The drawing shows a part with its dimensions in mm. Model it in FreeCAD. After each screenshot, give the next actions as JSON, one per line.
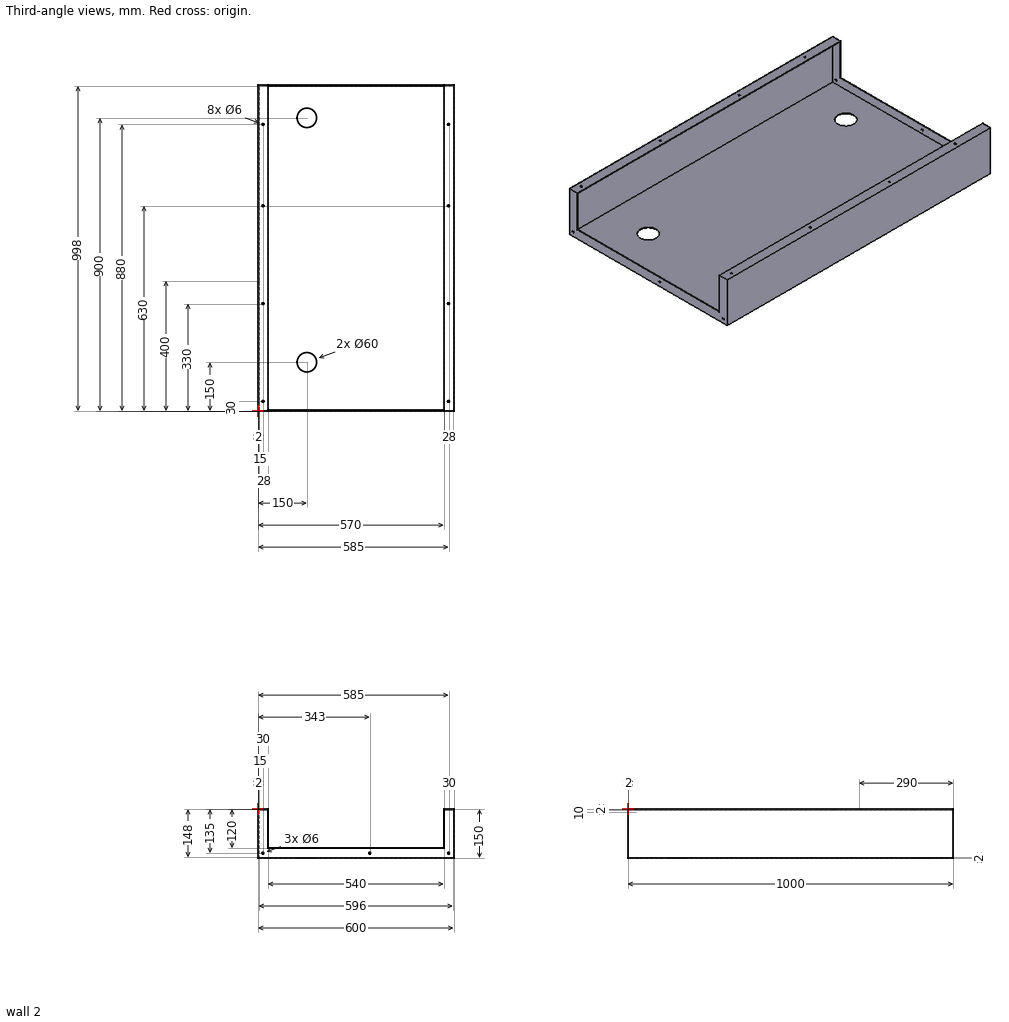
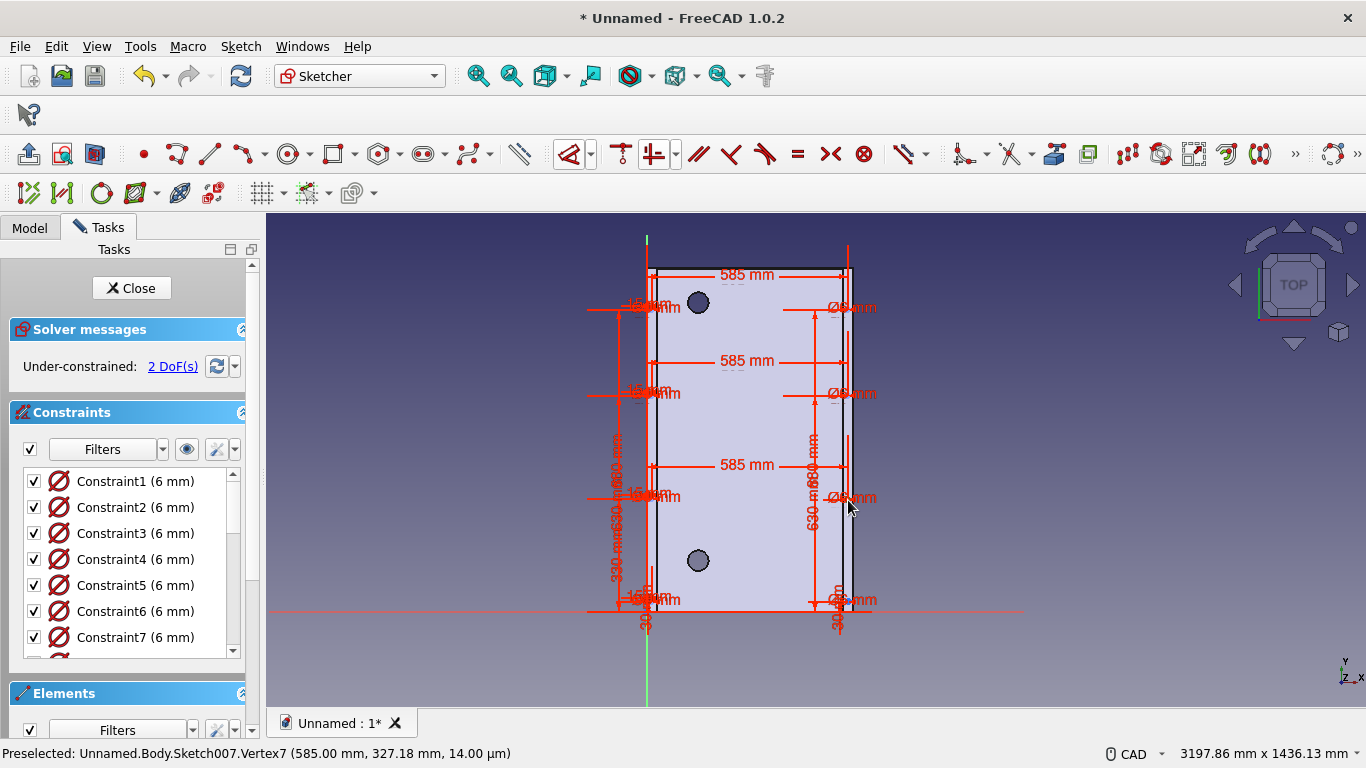
{"action": "key", "text": "i"}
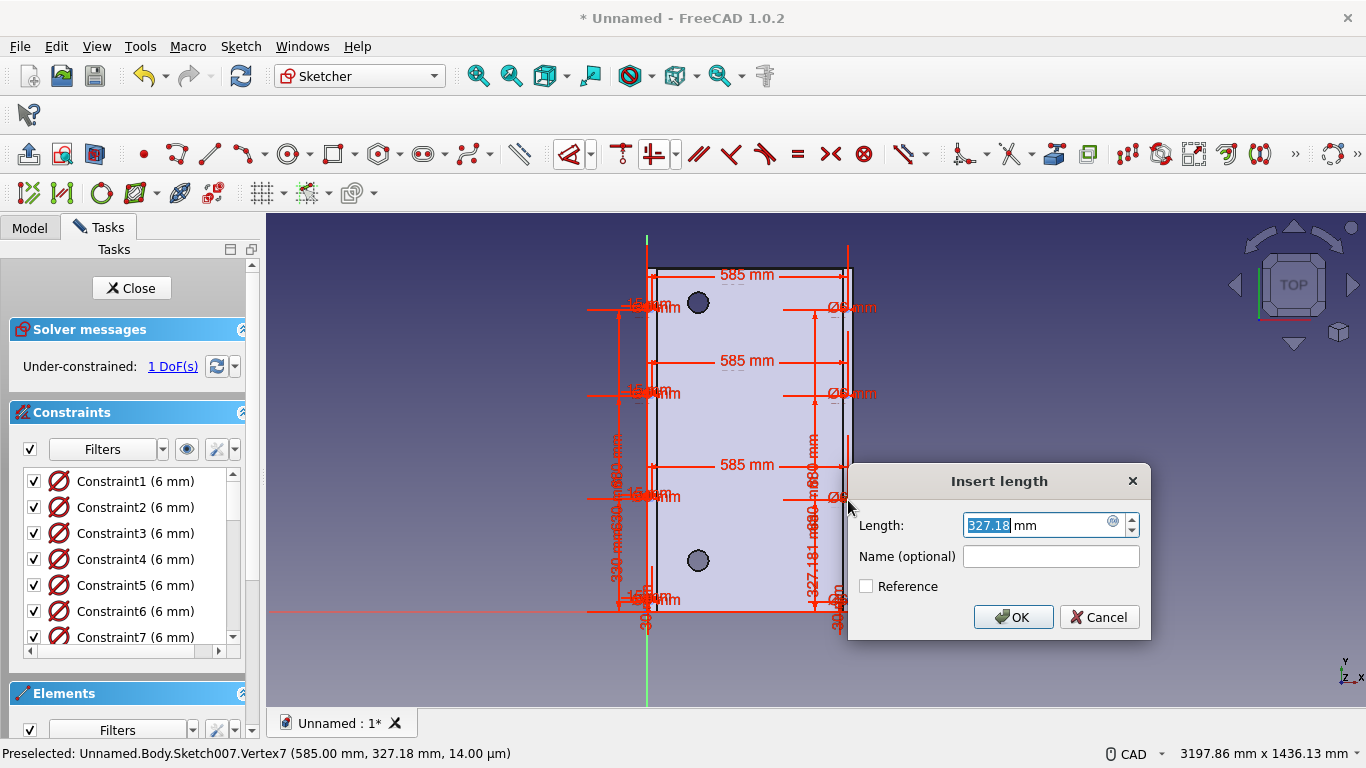
{"action": "type", "text": "330"}
{"action": "key", "text": "Return"}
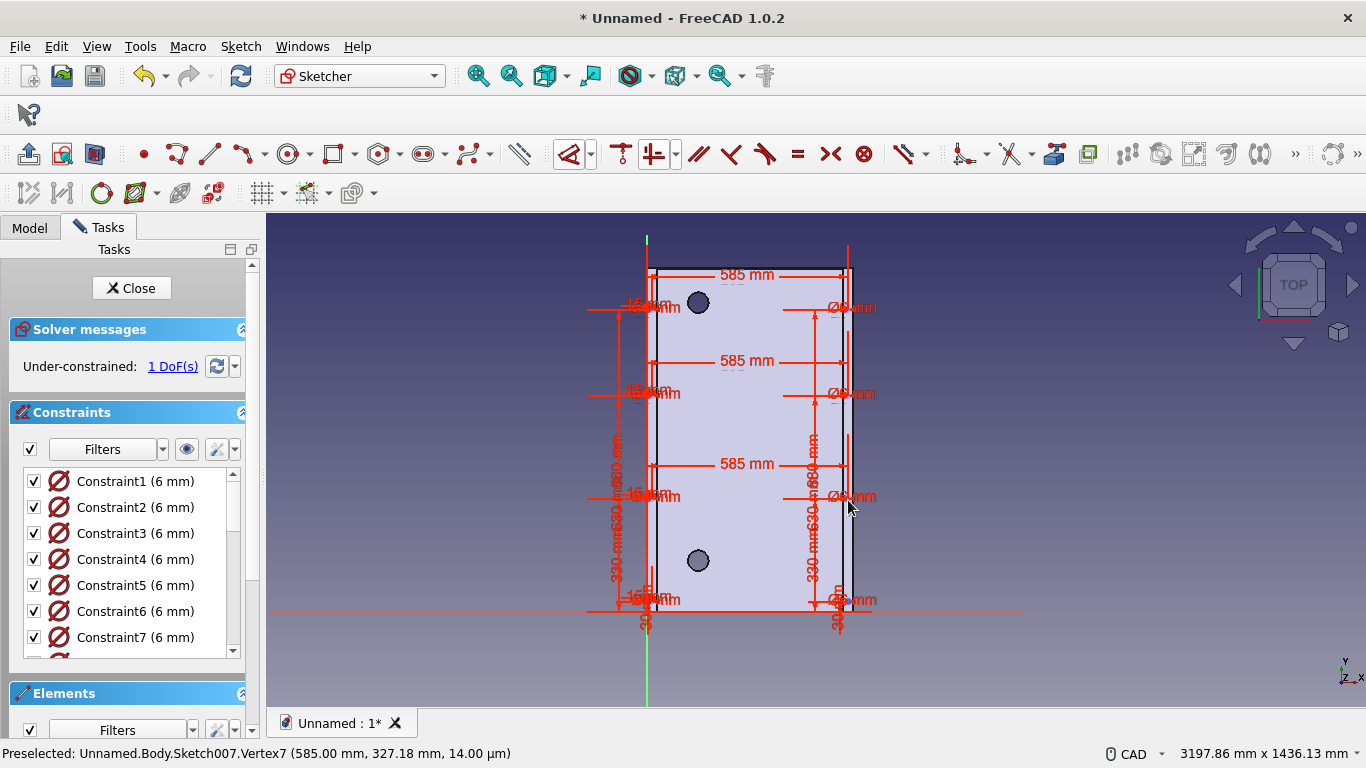
{"action": "left_click", "coordinate": [848, 602]}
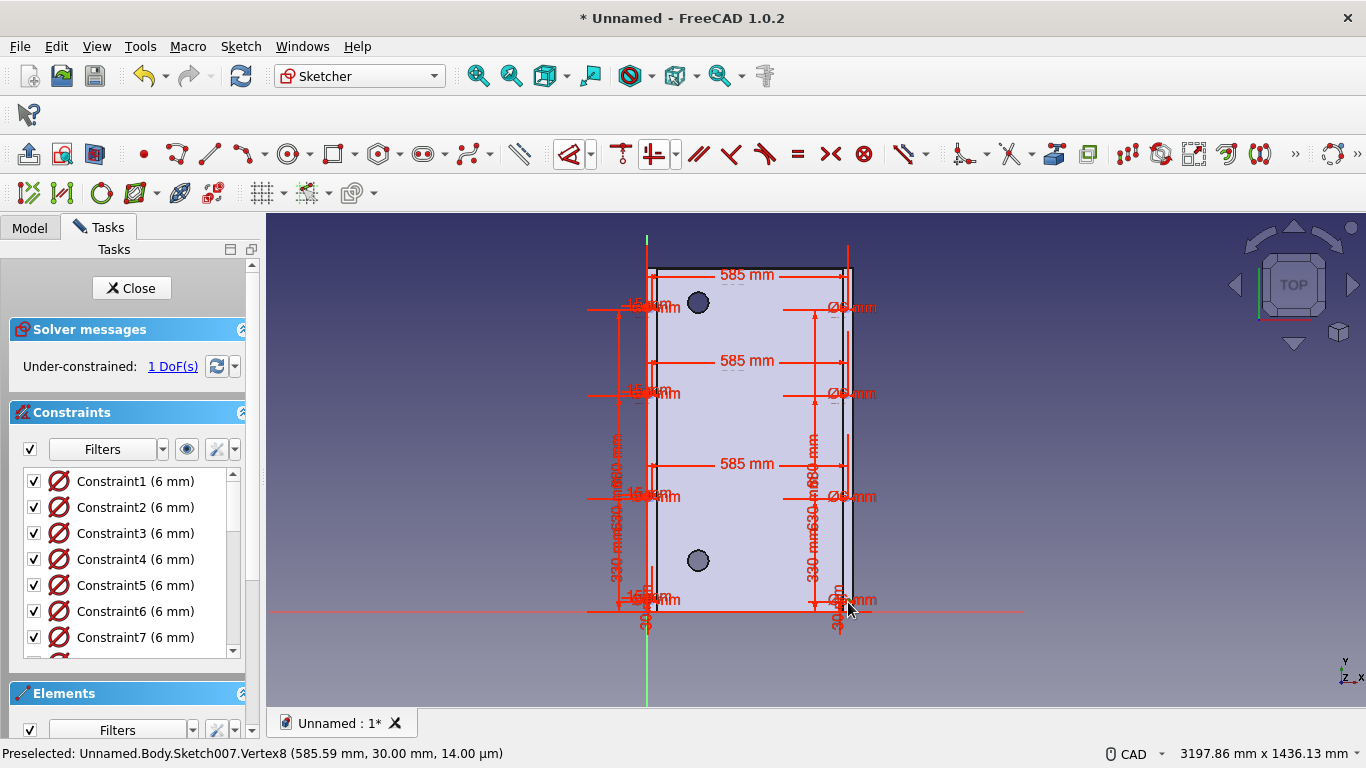
{"action": "left_click", "coordinate": [590, 154]}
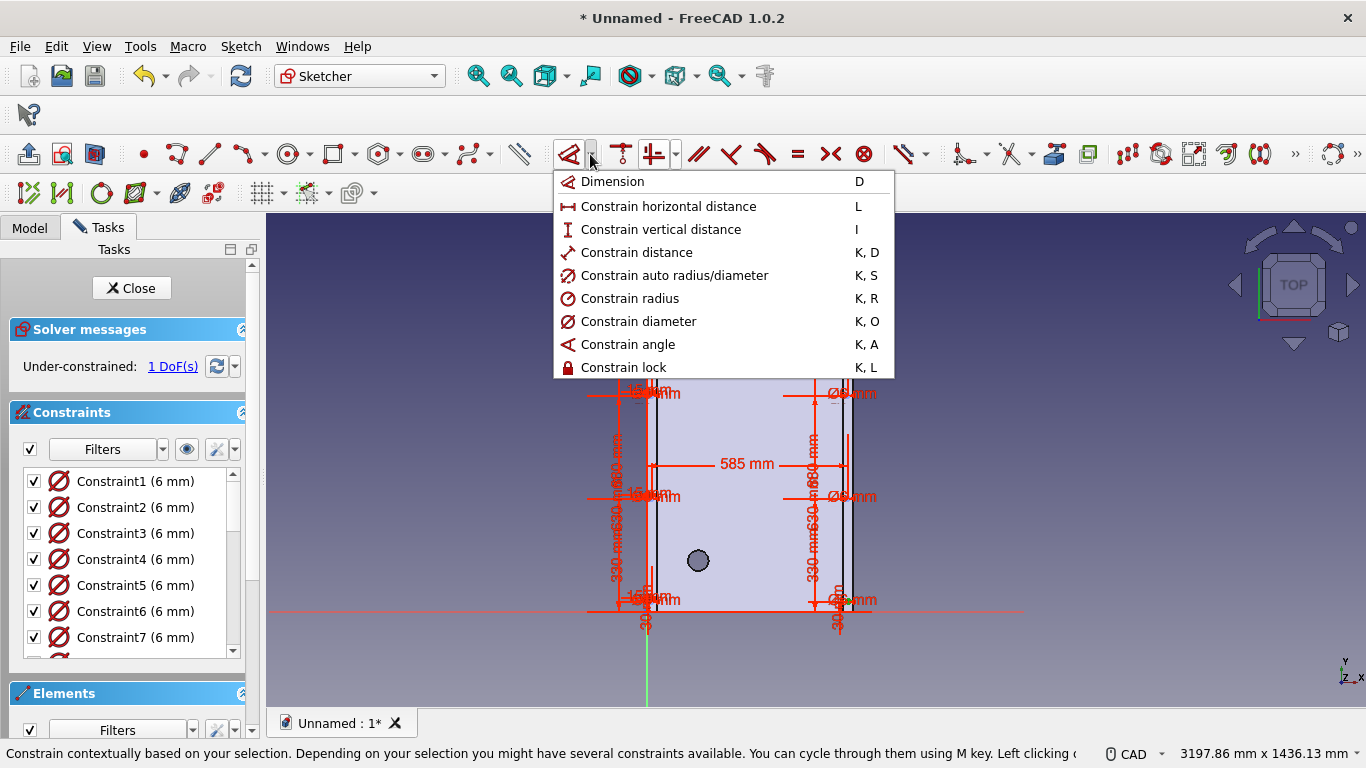
{"action": "left_click", "coordinate": [724, 206]}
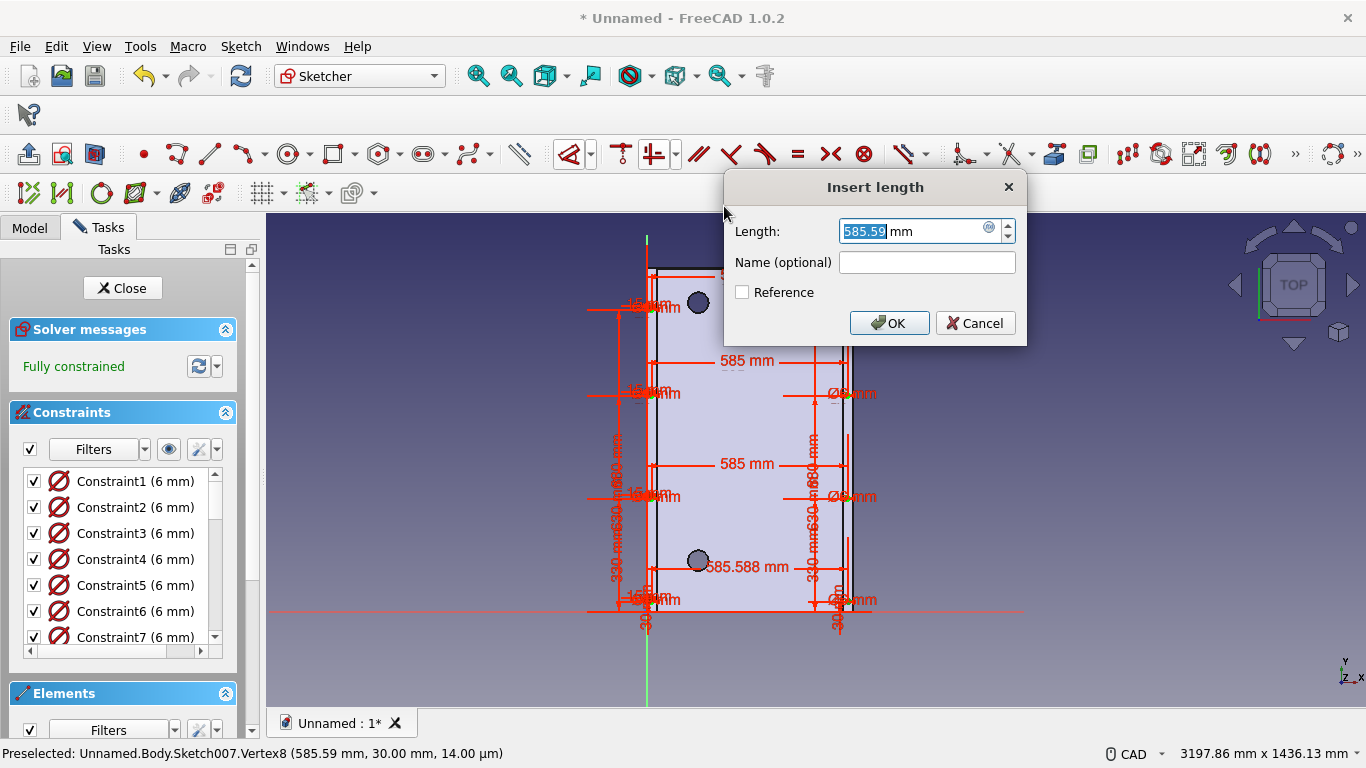
{"action": "type", "text": "585"}
{"action": "key", "text": "Return"}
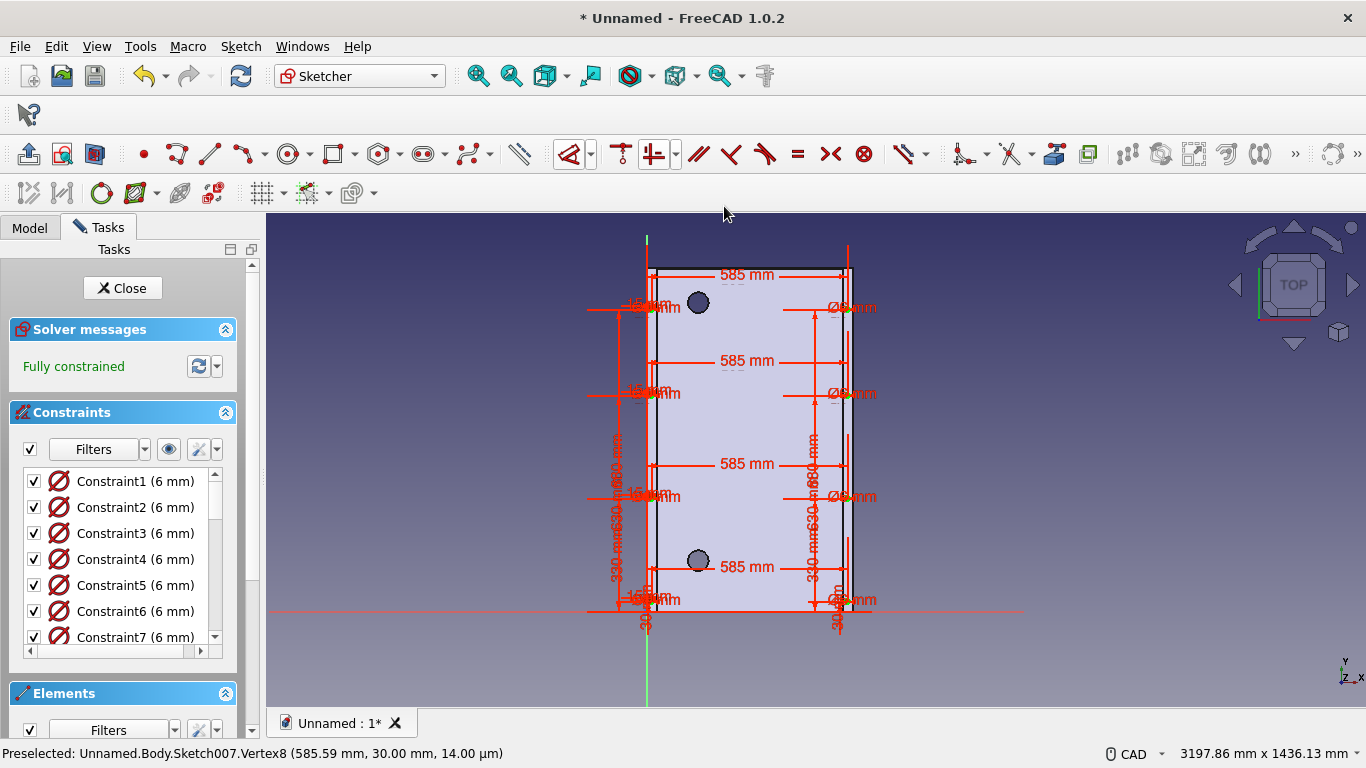
{"action": "left_click", "coordinate": [123, 288]}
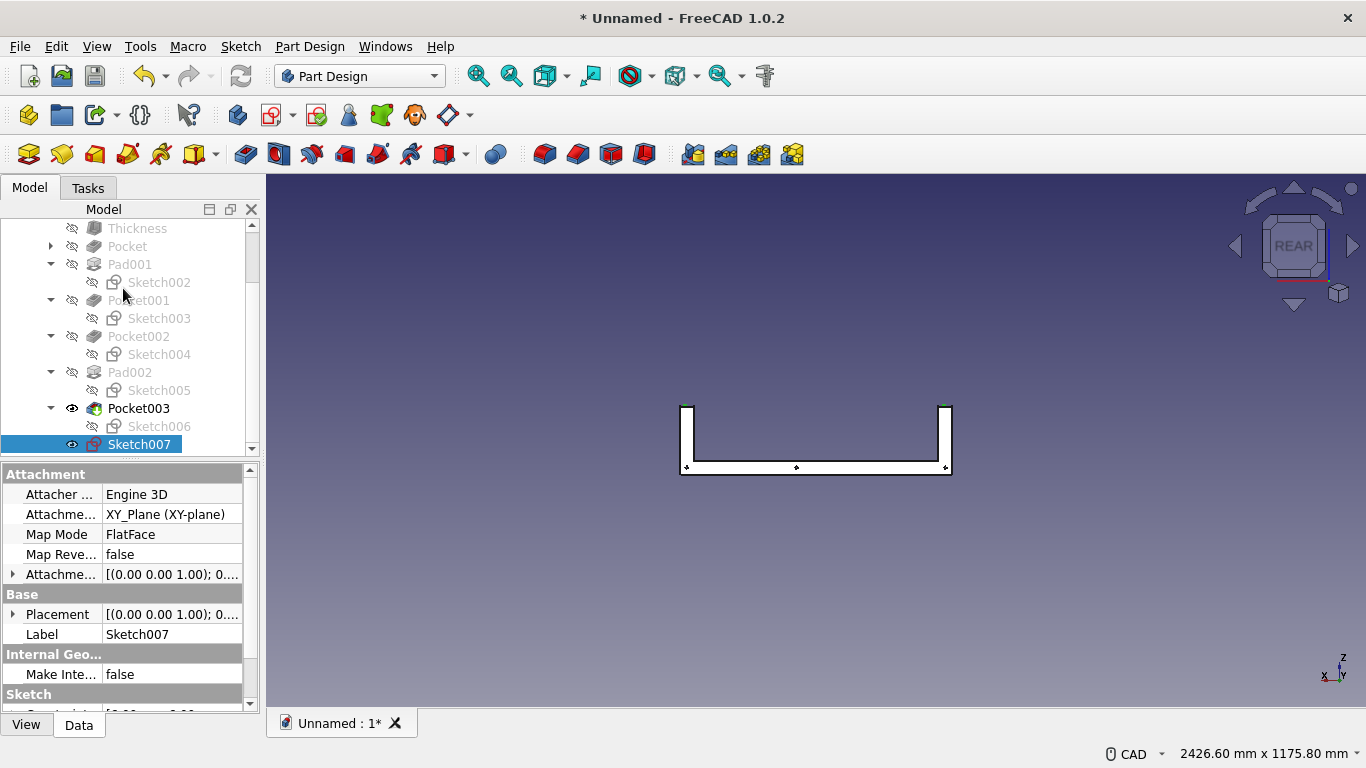
{"action": "left_click", "coordinate": [246, 154]}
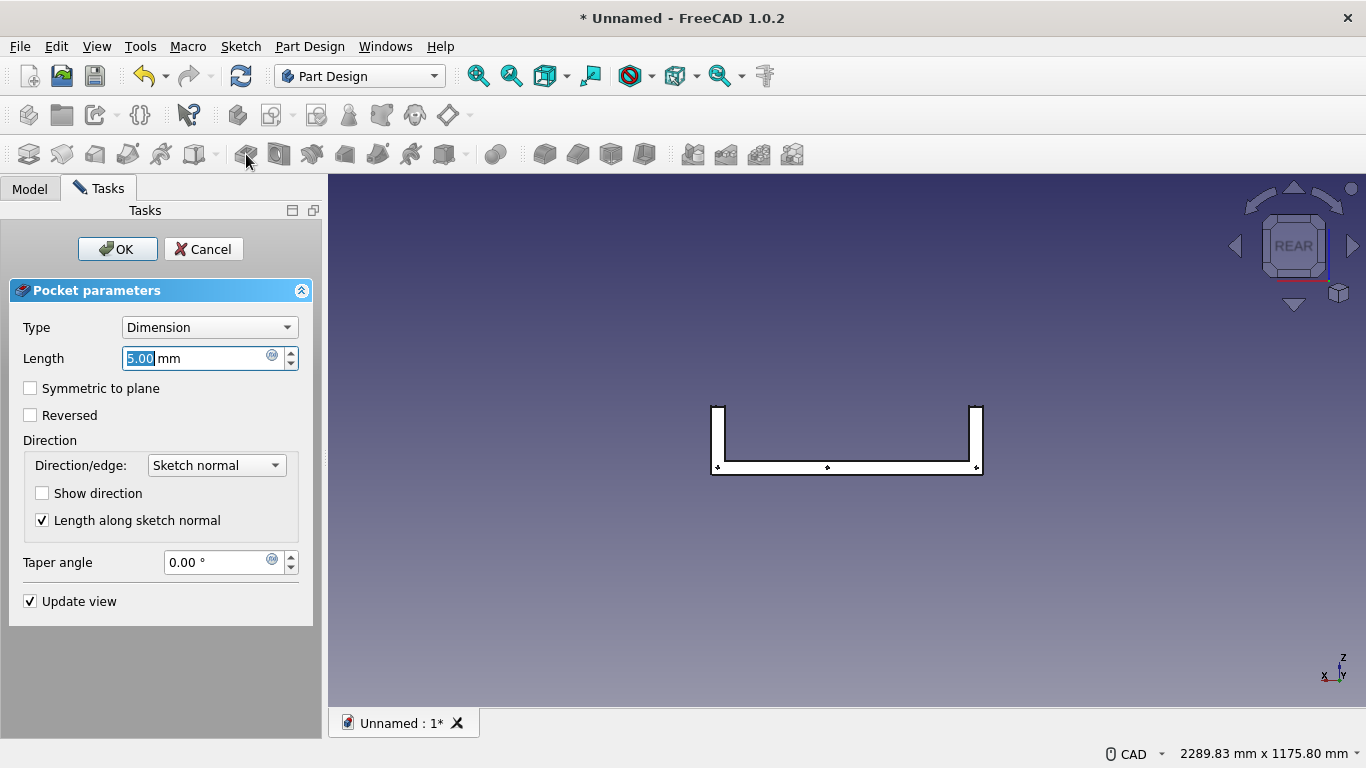
{"action": "type", "text": "10"}
{"action": "key", "text": "Tab"}